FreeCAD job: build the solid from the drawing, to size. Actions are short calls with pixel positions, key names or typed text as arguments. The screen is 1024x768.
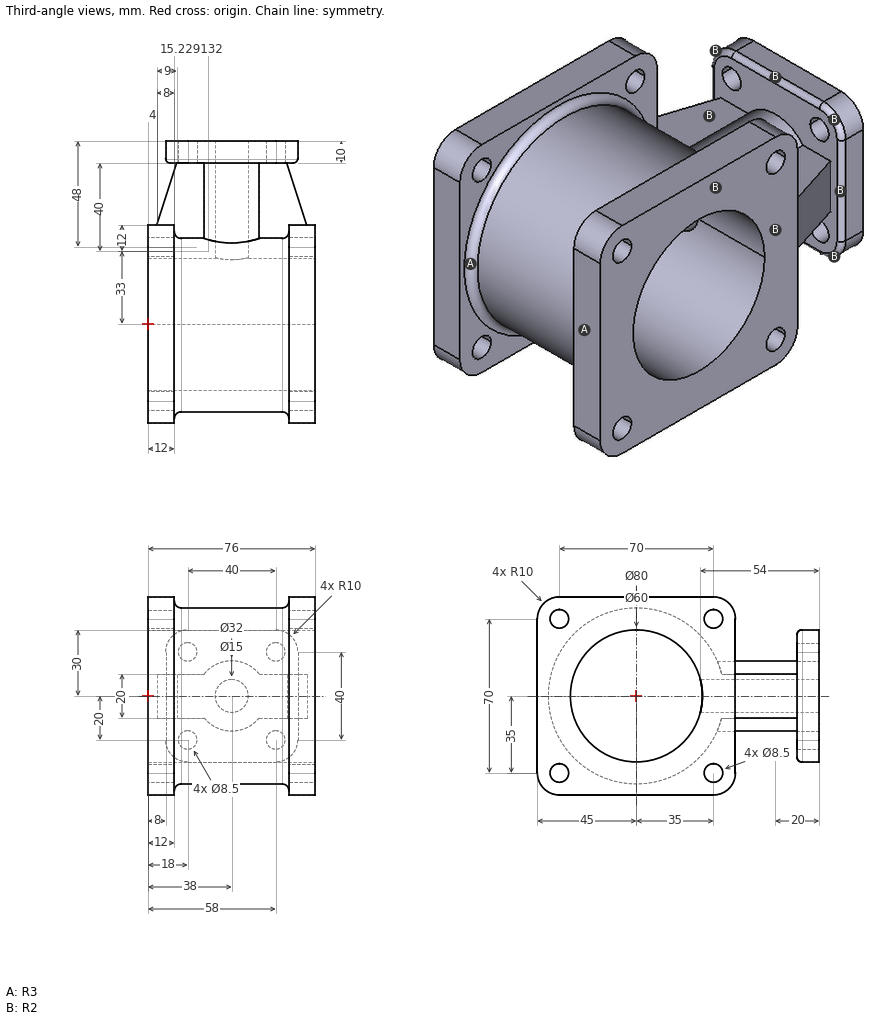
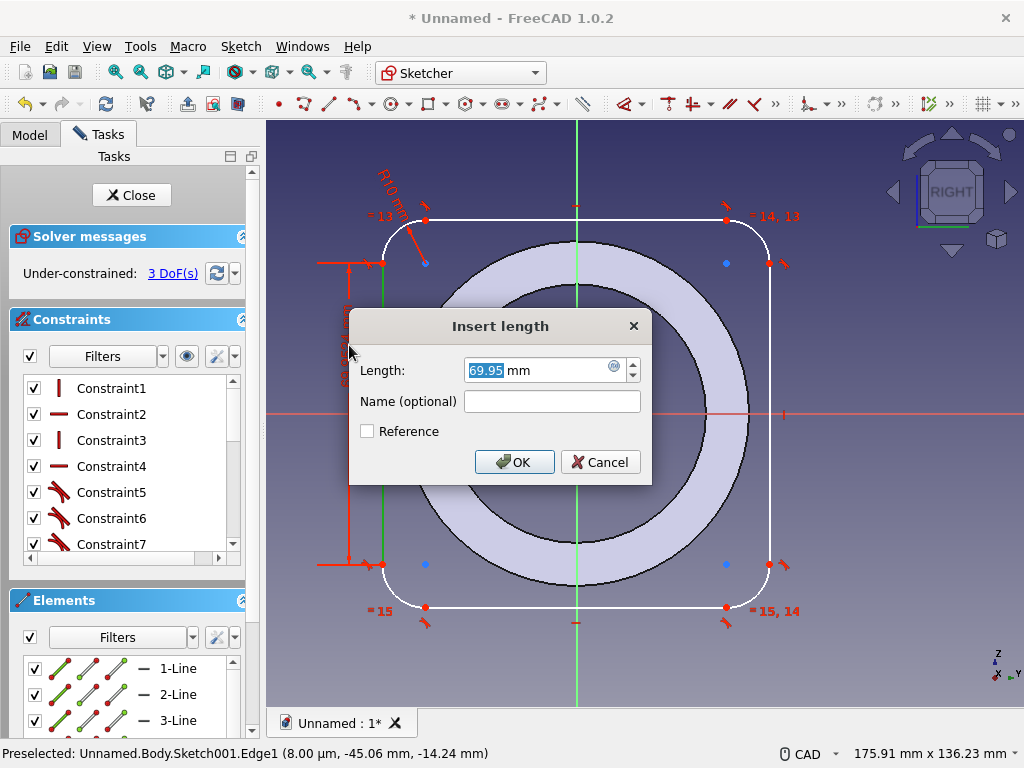
text(70)
key(Return)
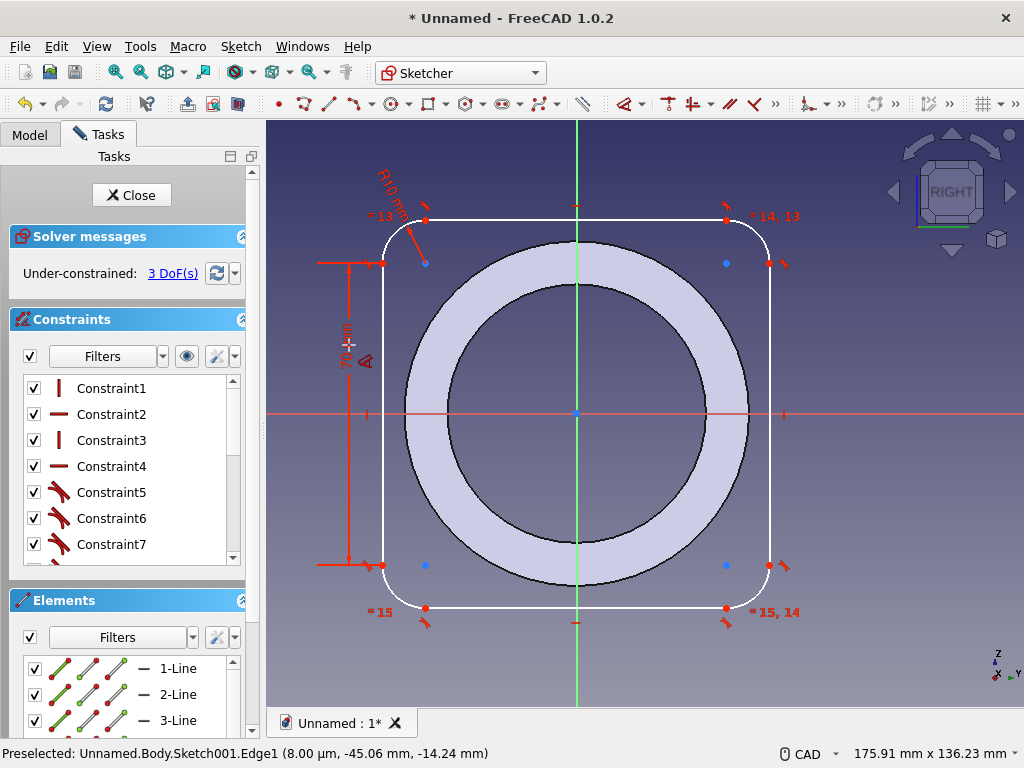
click(516, 220)
click(507, 186)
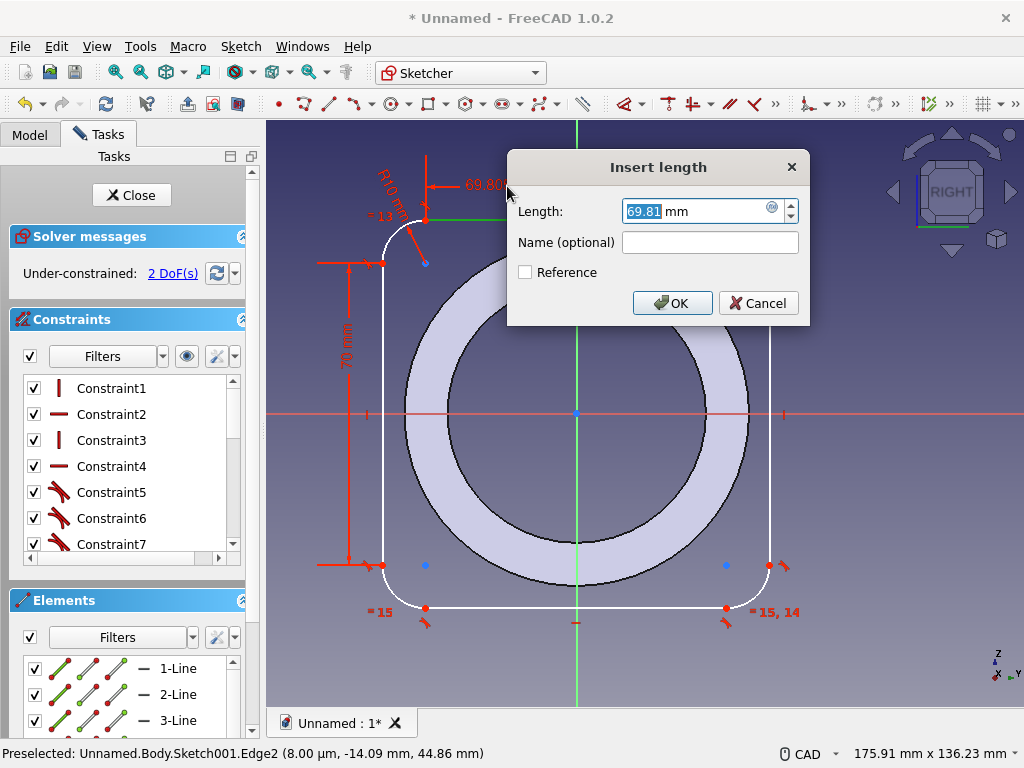
text(70)
key(Return)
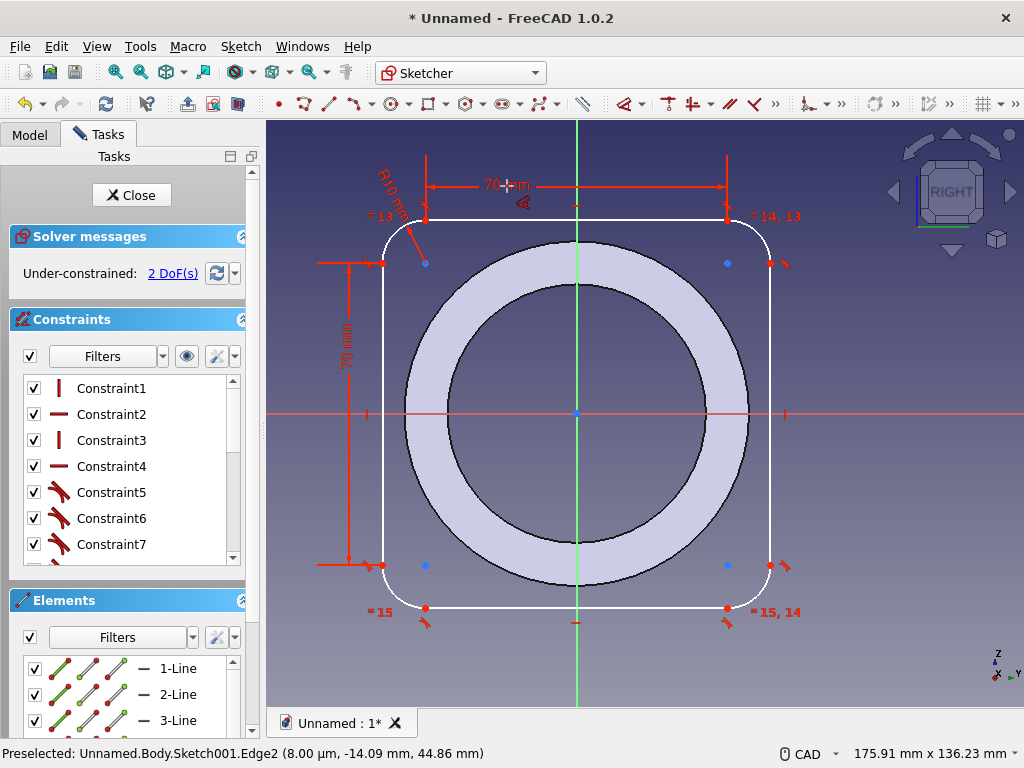
click(383, 565)
click(480, 380)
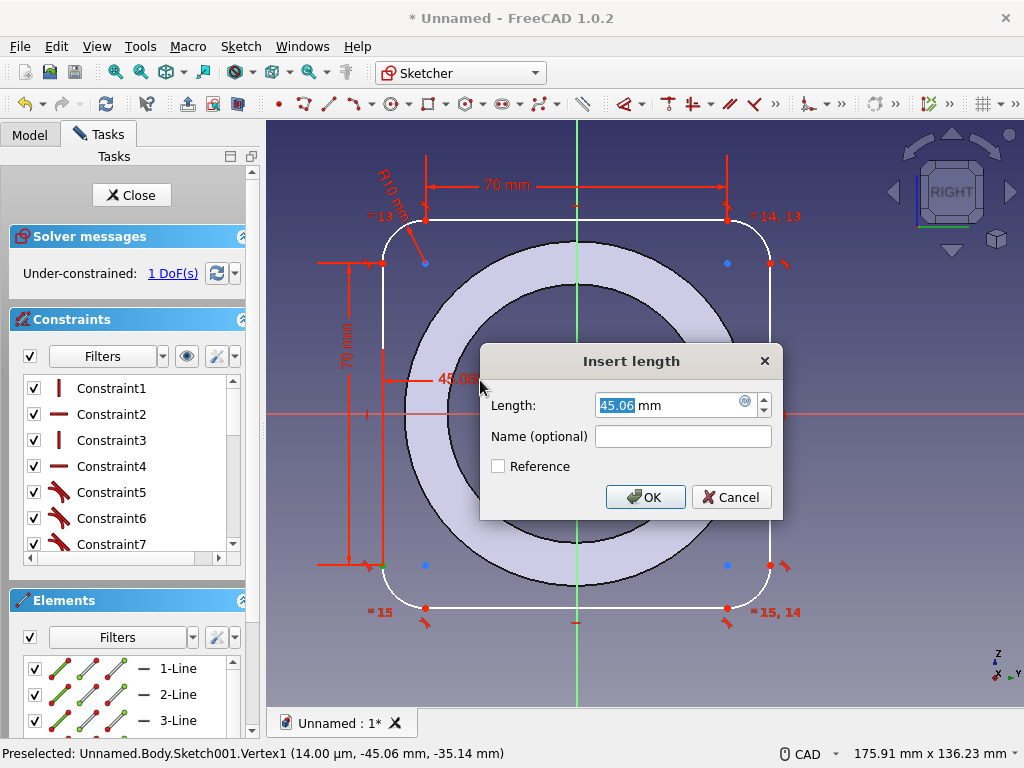
text(45)
key(Return)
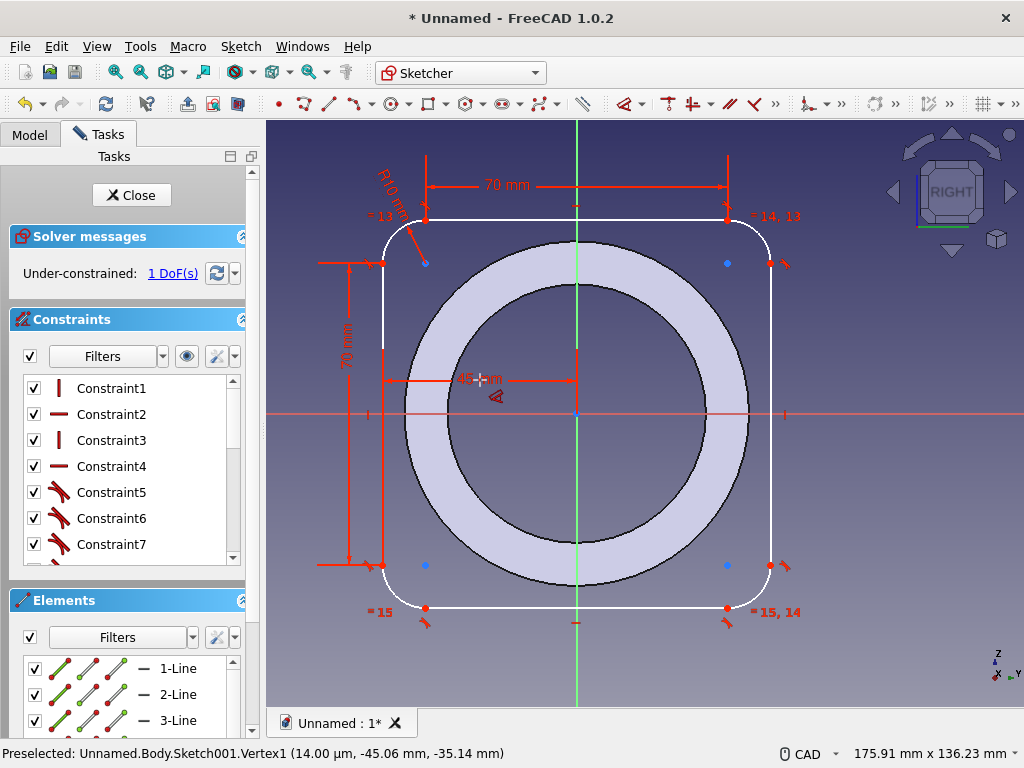
click(383, 565)
click(349, 489)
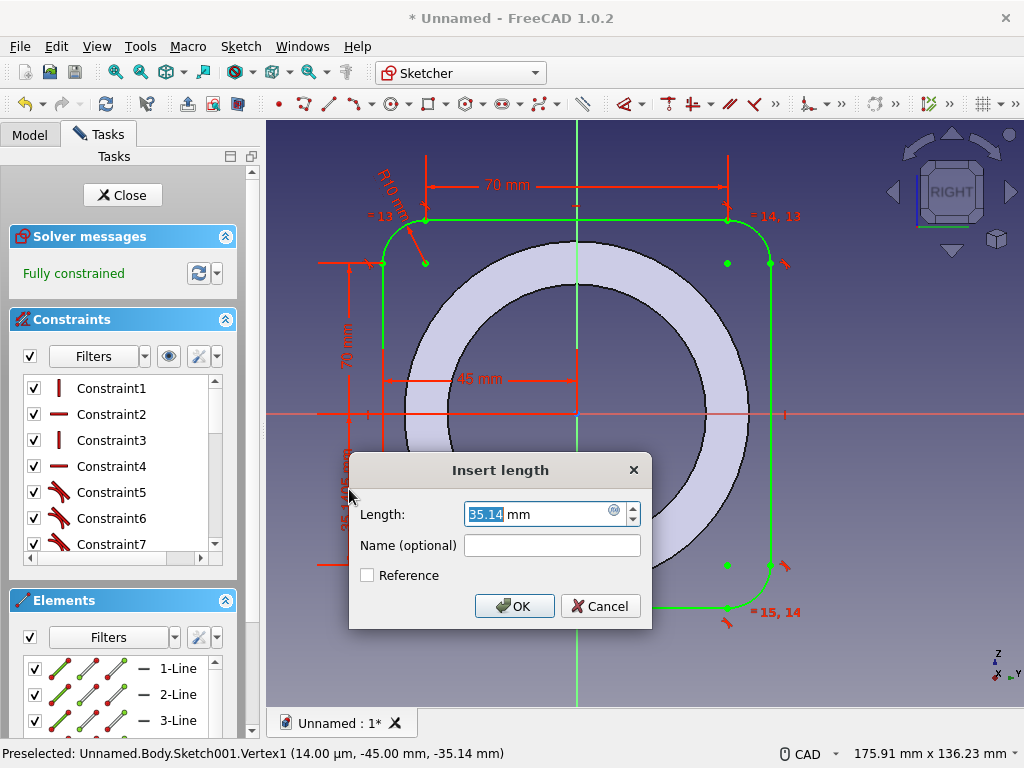
text(35)
key(Return)
key(Escape)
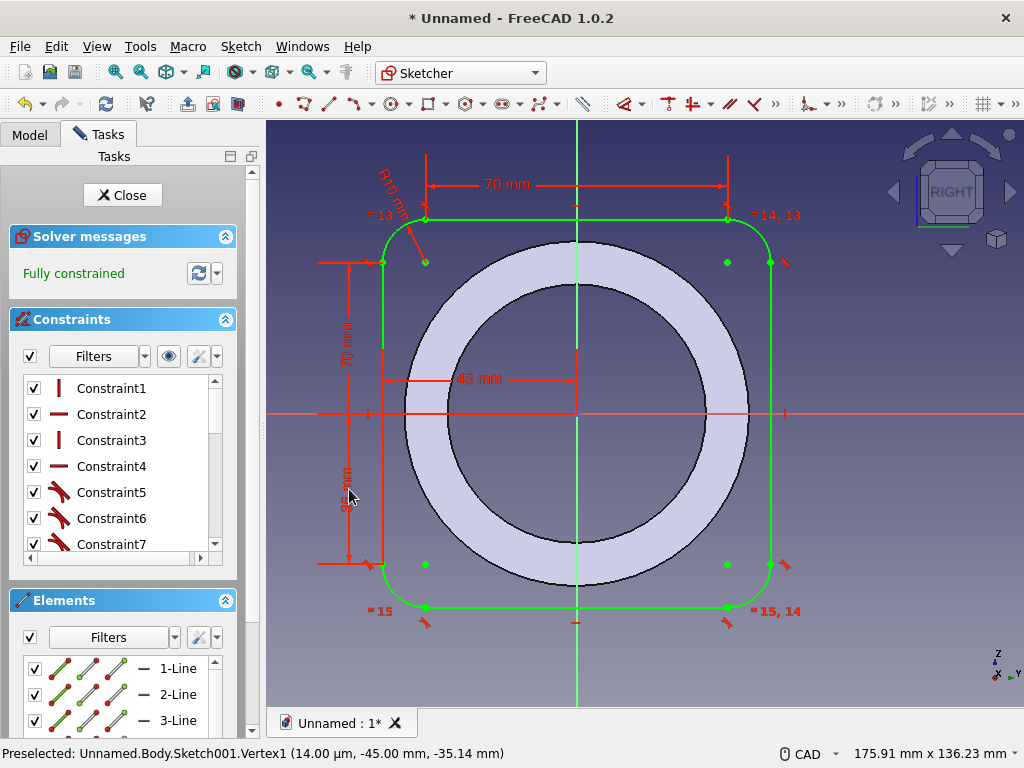
click(123, 195)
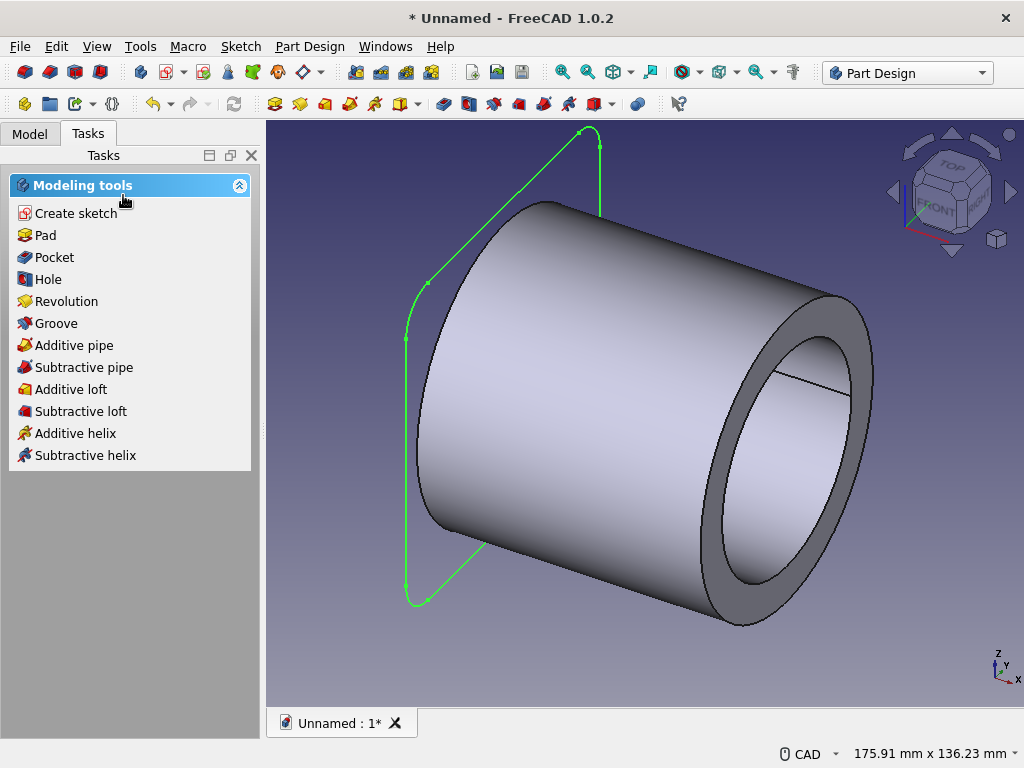
click(275, 104)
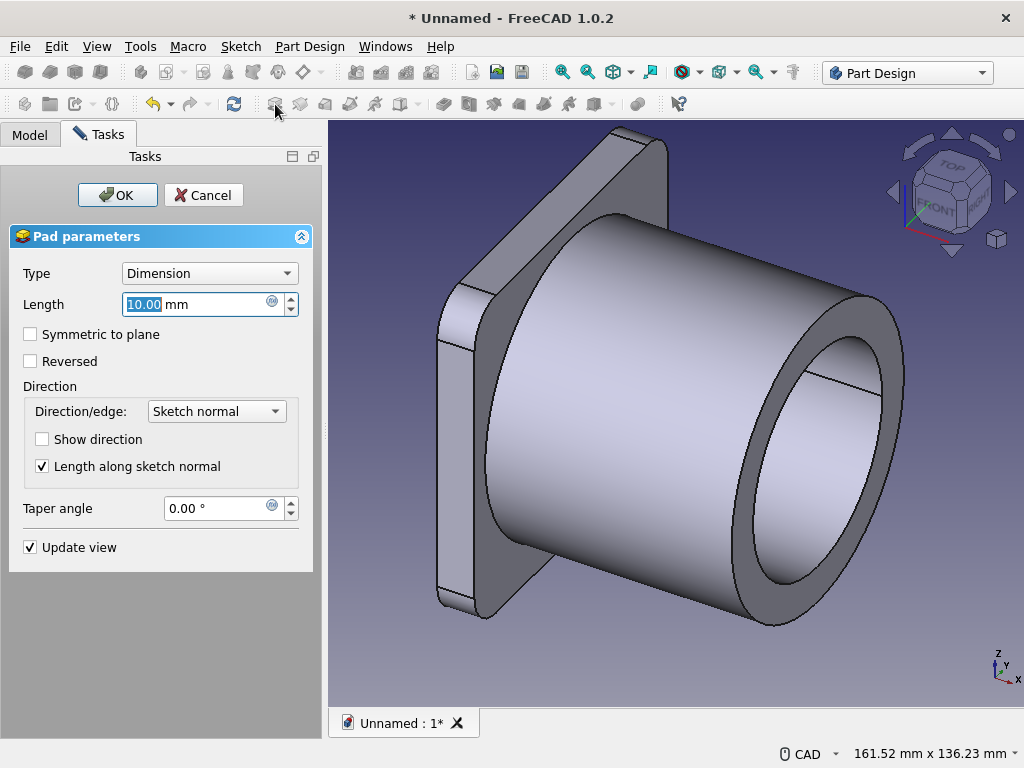
text(12)
key(Tab)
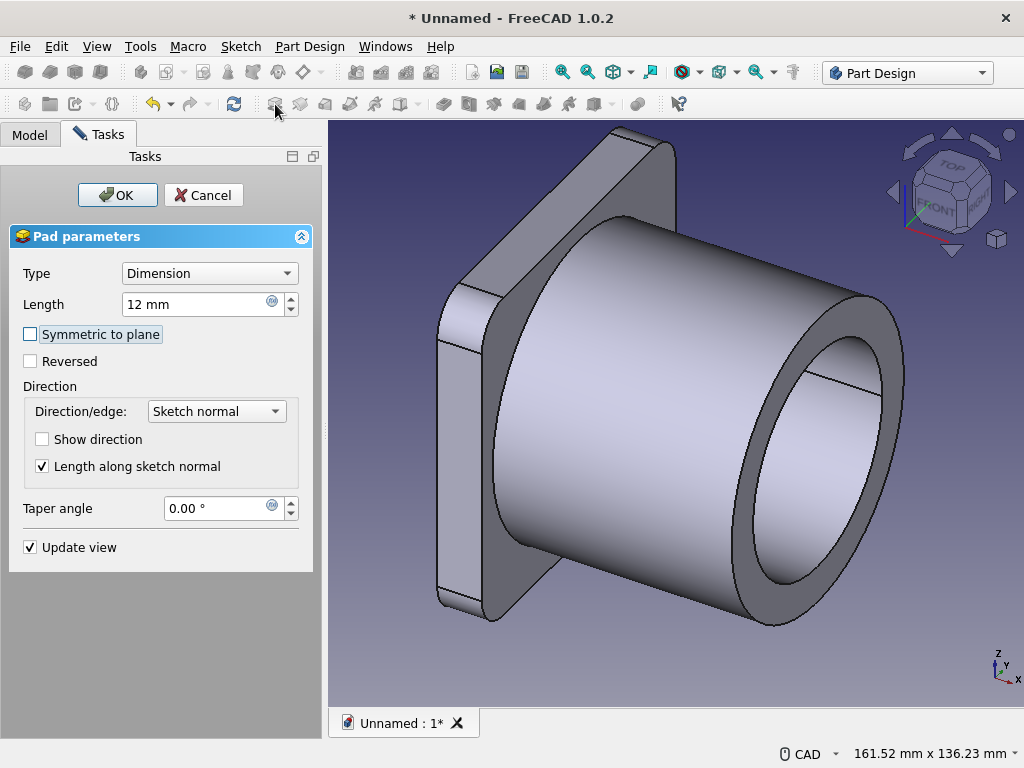
click(118, 195)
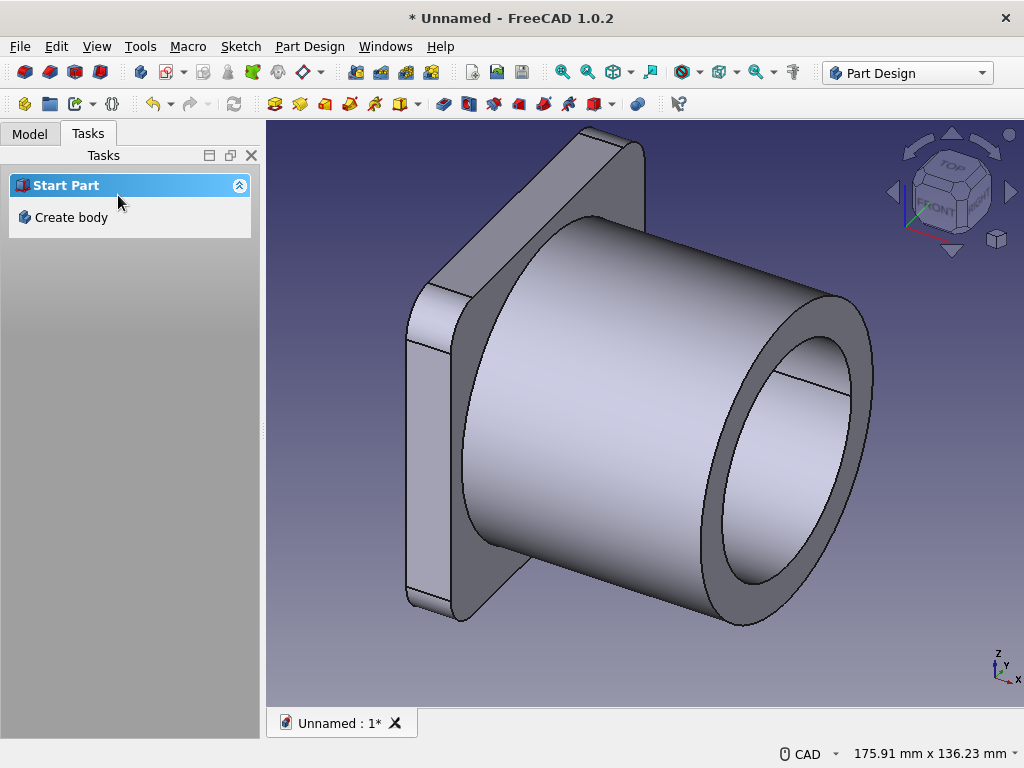
key(v)
key(f)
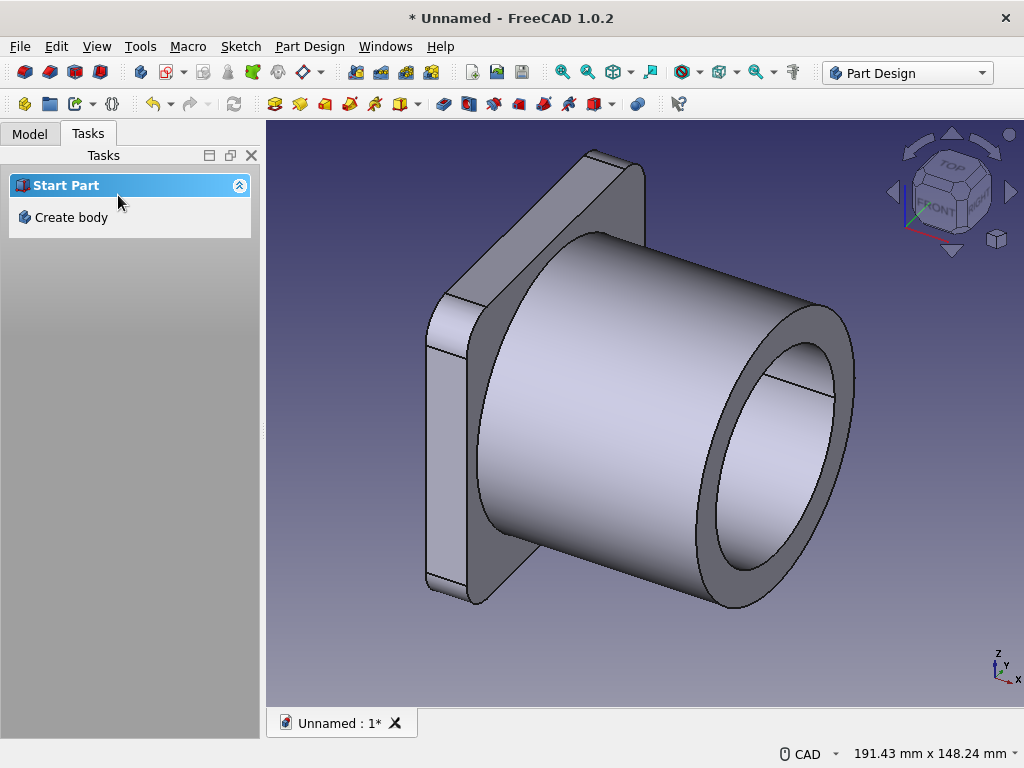
key(6)